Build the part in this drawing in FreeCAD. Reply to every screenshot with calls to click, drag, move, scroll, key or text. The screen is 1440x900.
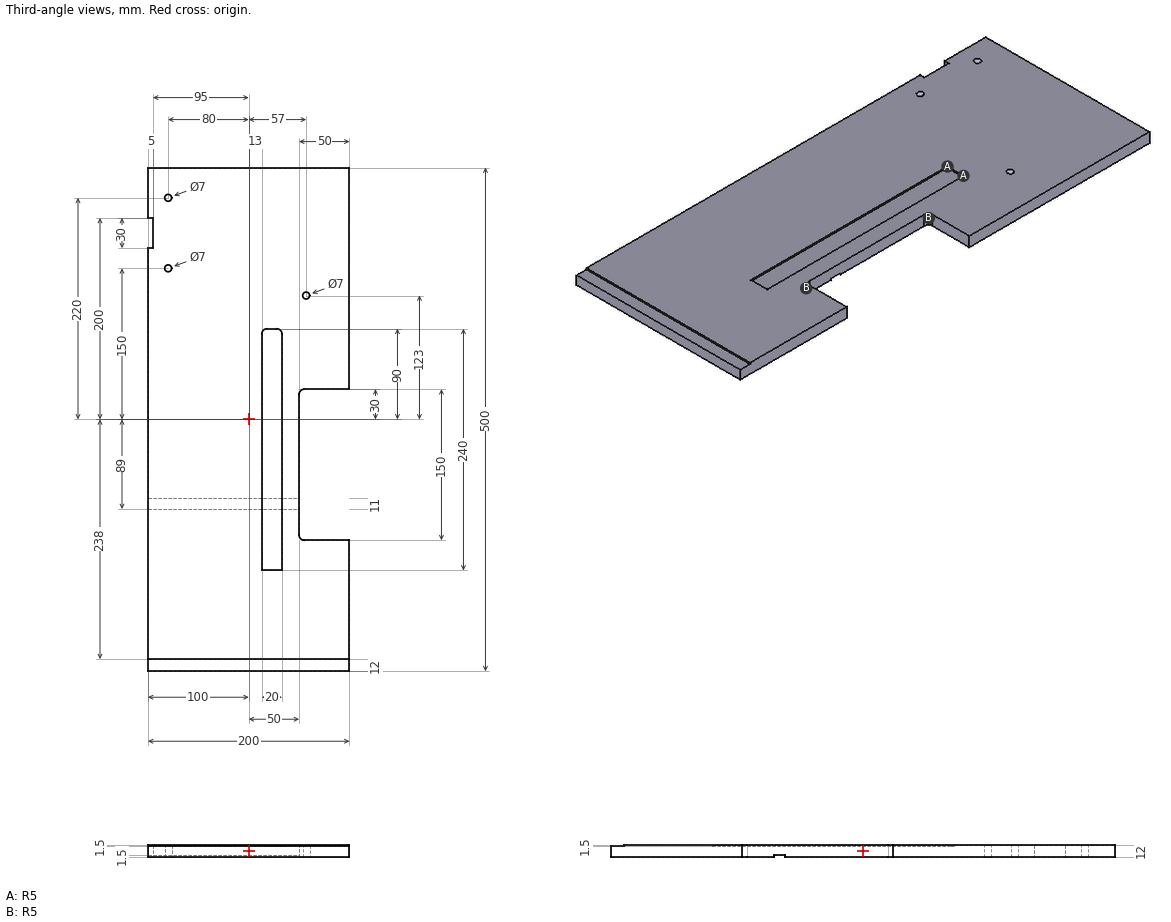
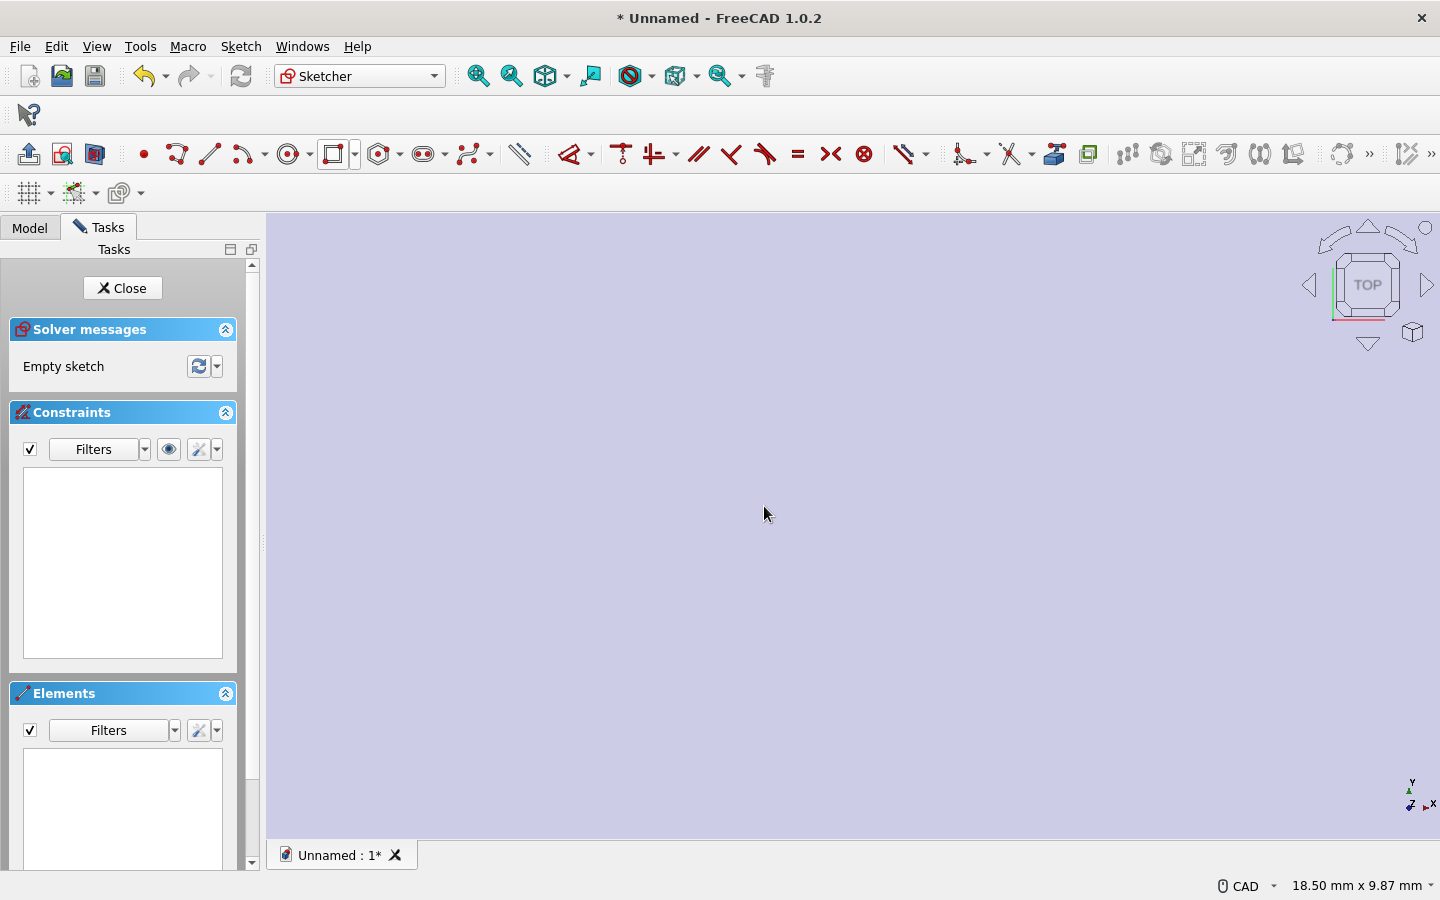
key(g)
key(c)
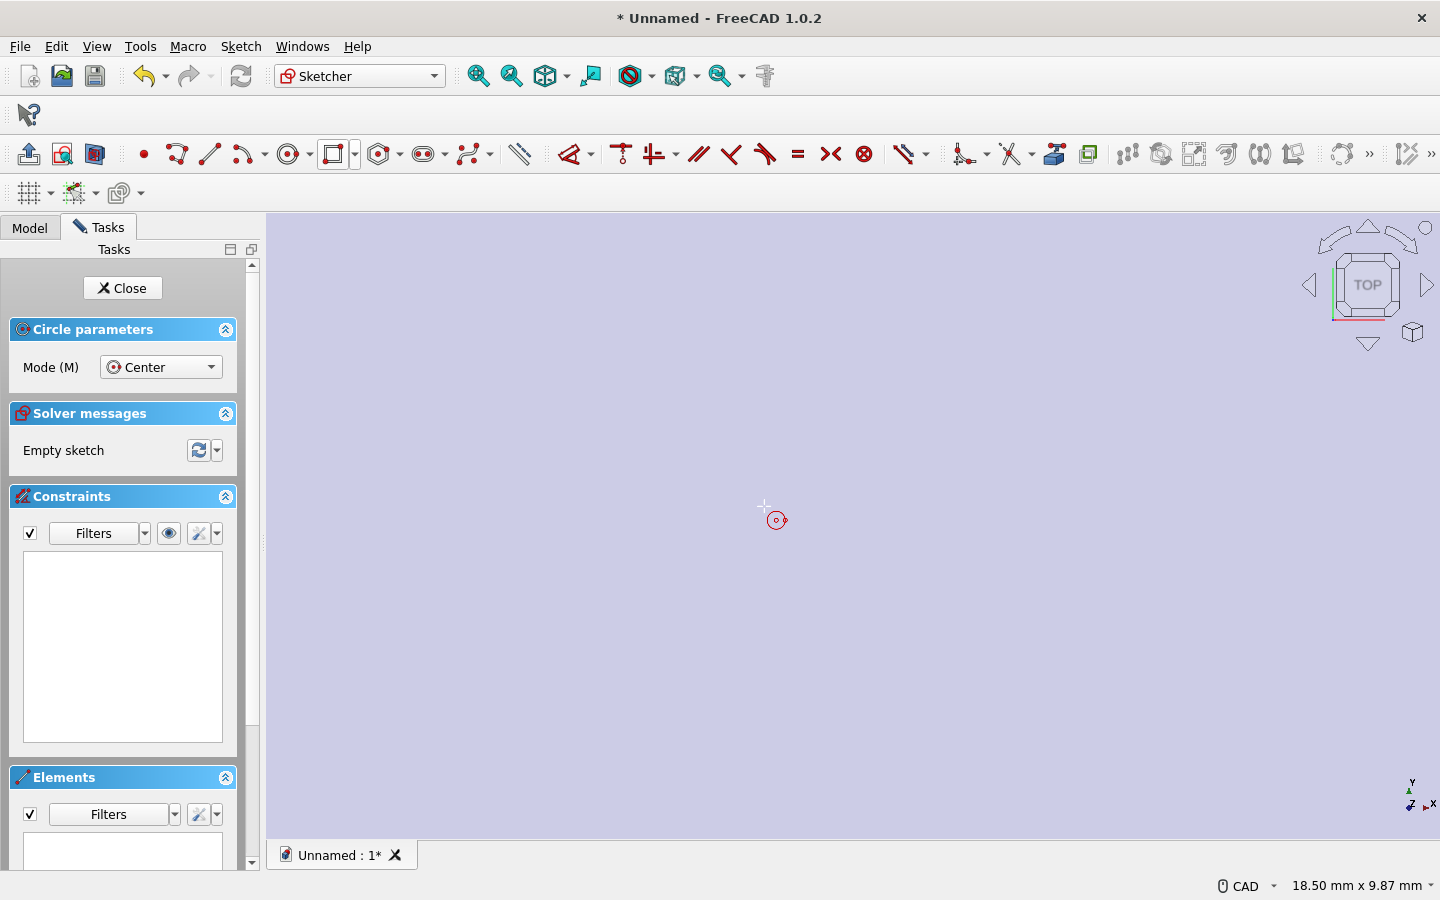
click(784, 525)
move(941, 368)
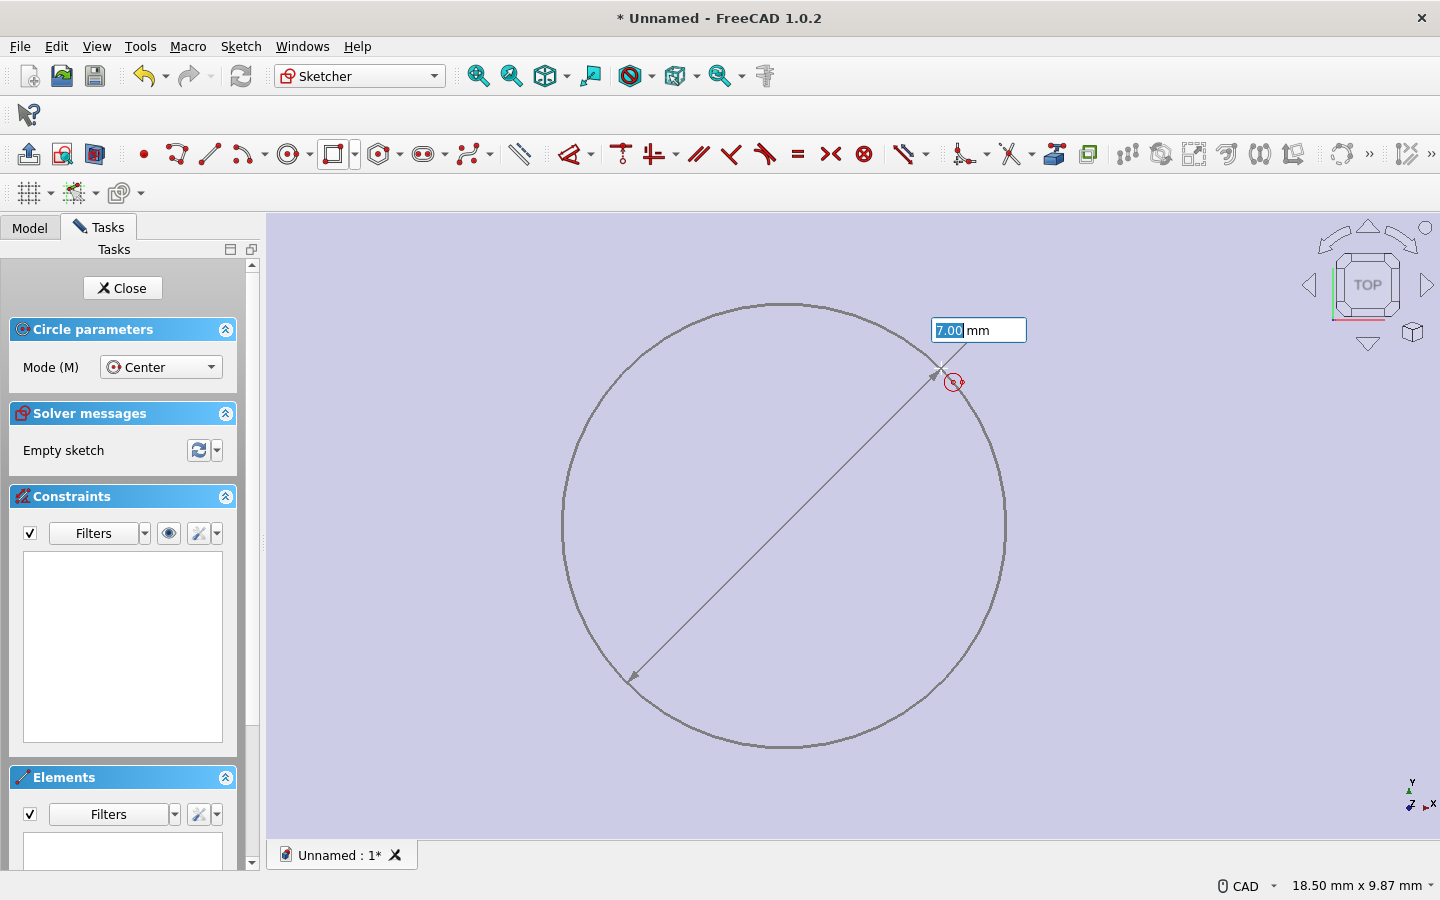
text(7)
key(Return)
key(Escape)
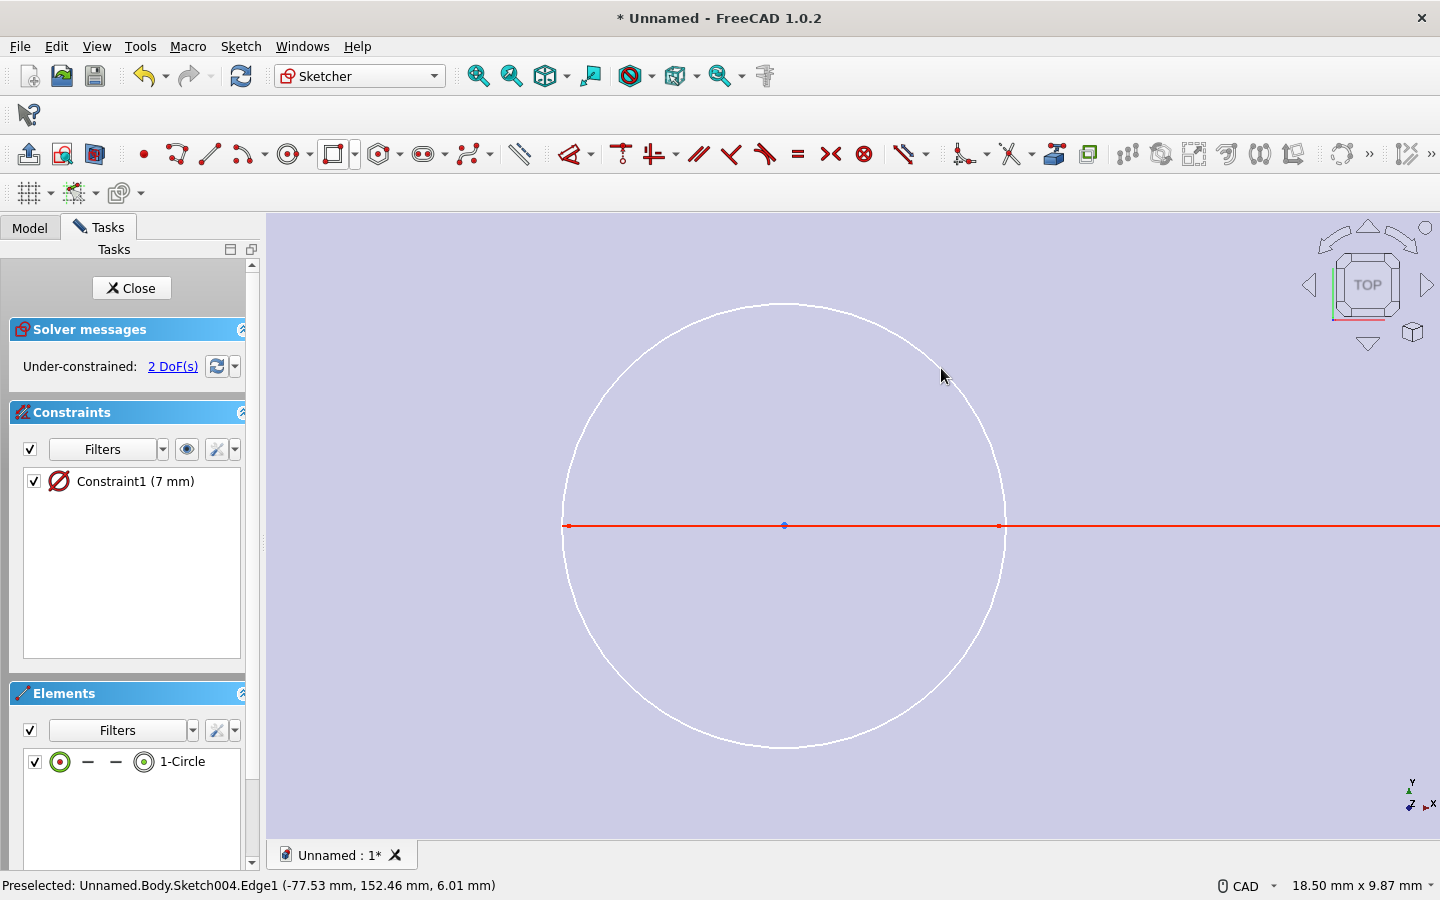
click(568, 154)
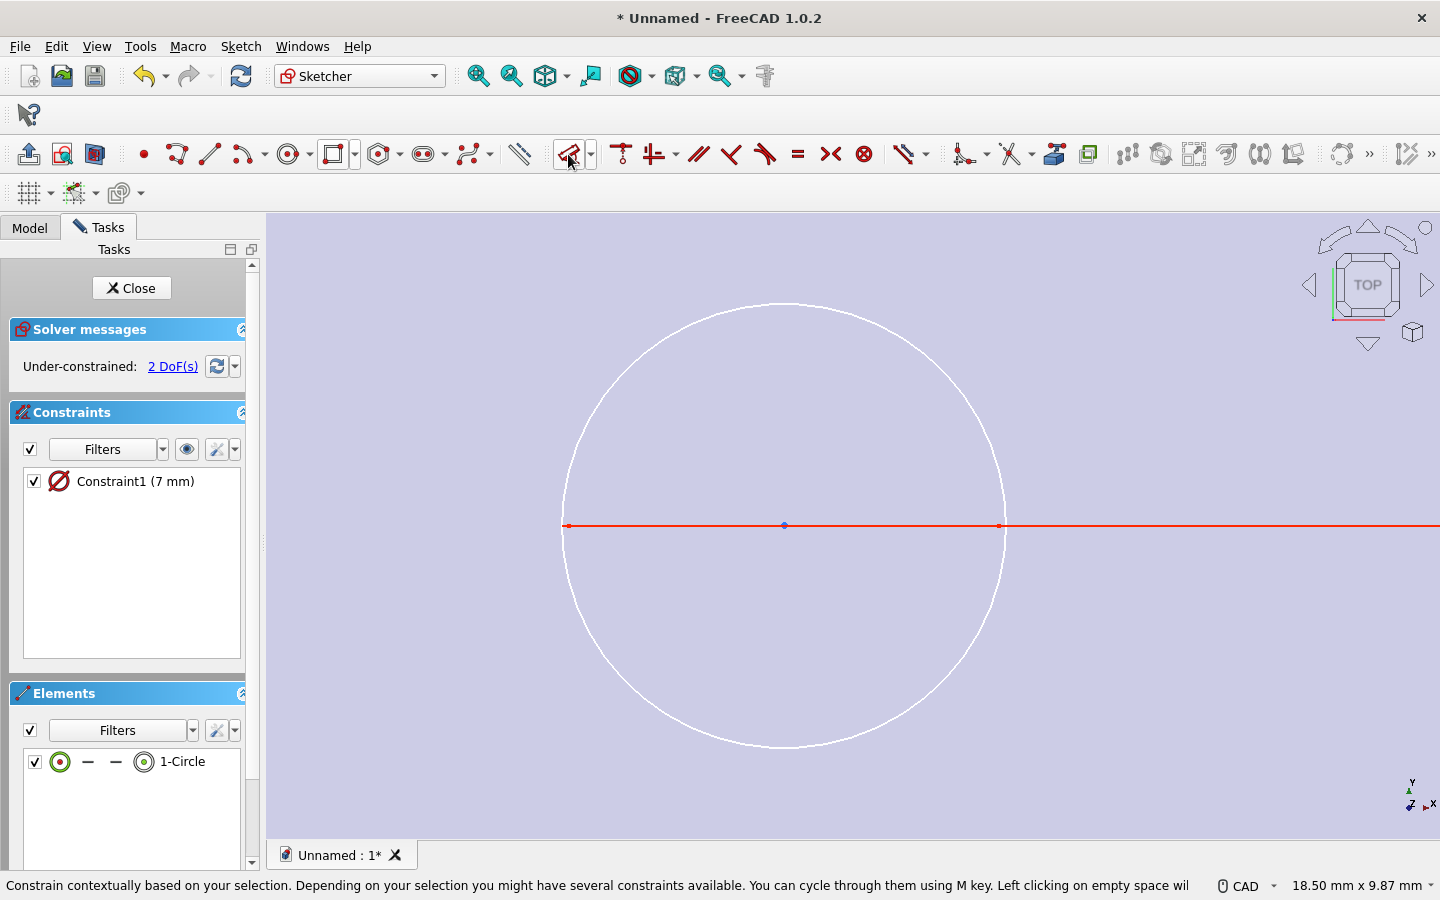
click(784, 526)
click(1030, 492)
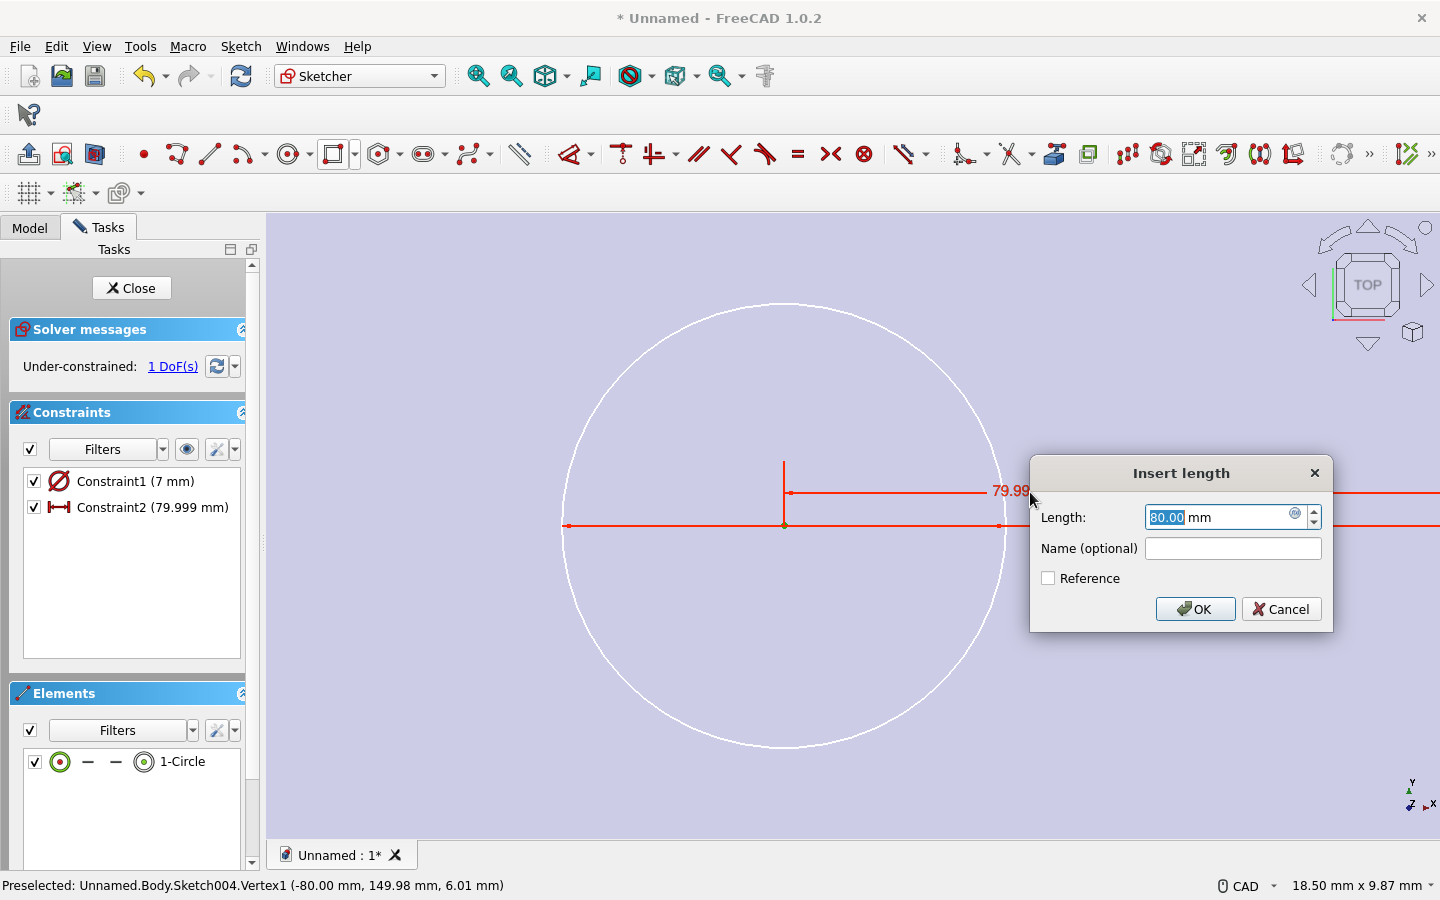
text(80)
key(Return)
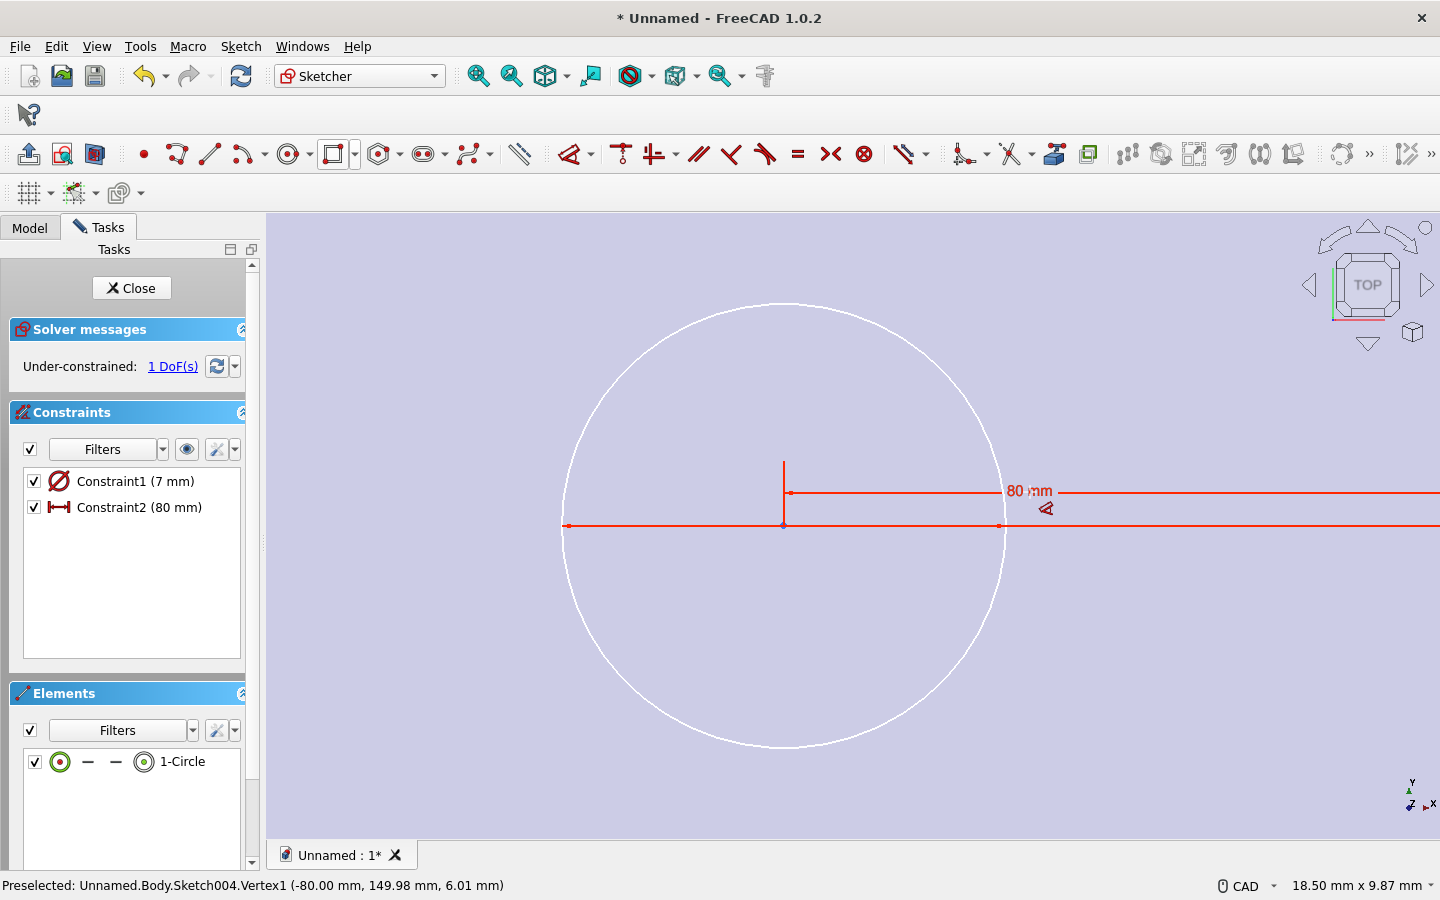
click(784, 526)
click(750, 668)